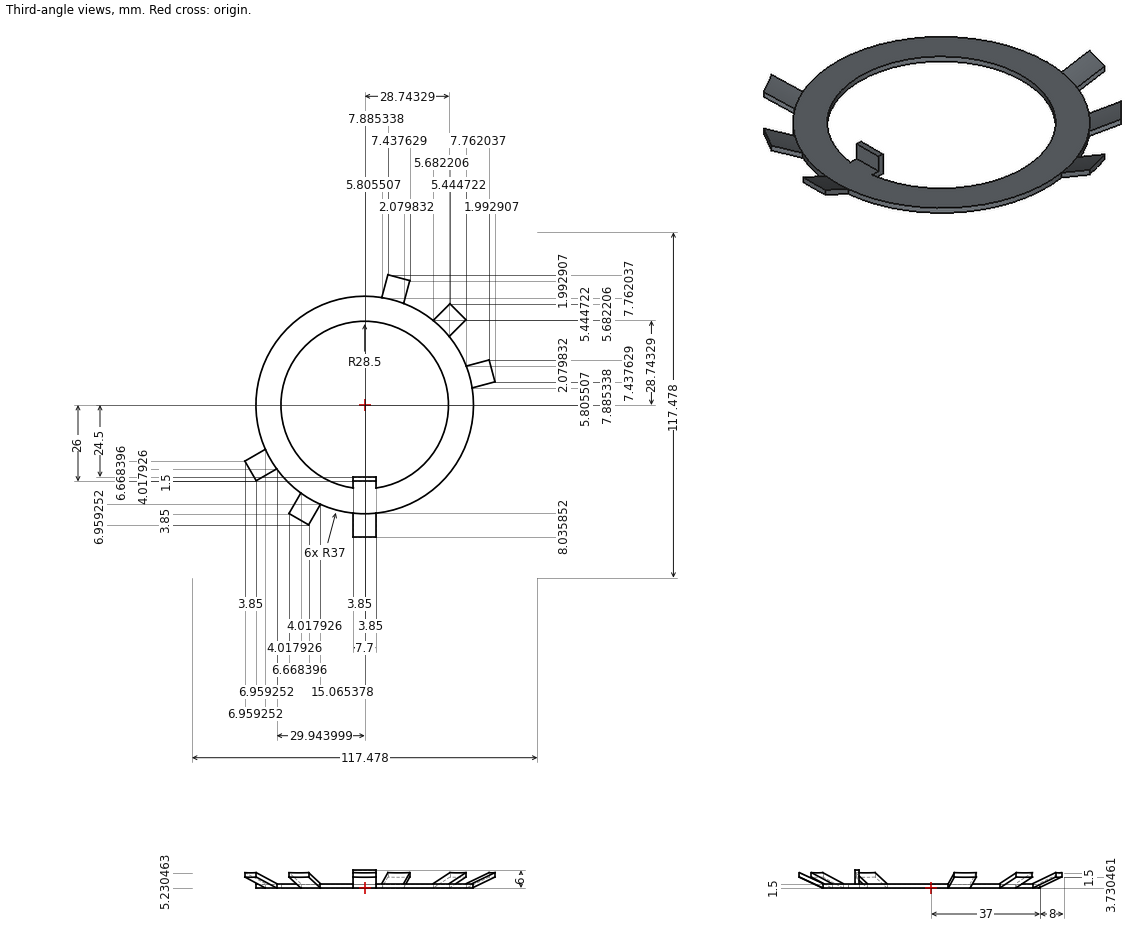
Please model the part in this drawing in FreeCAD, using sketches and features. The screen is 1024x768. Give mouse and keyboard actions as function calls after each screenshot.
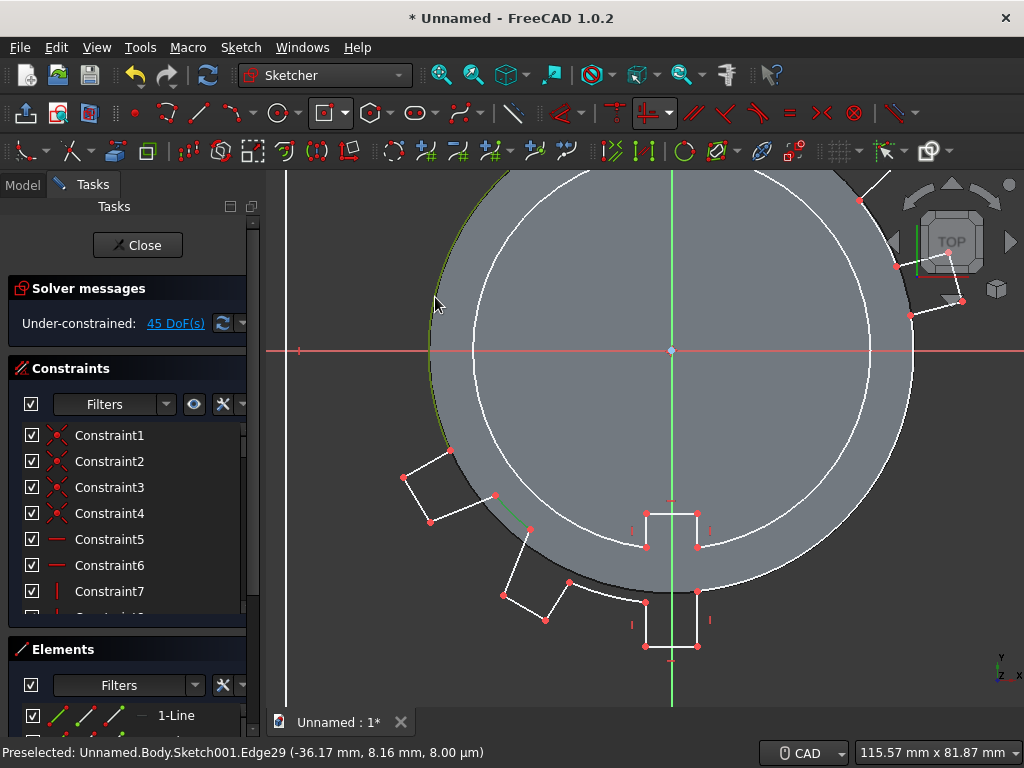
scroll(499, 510, down, 4)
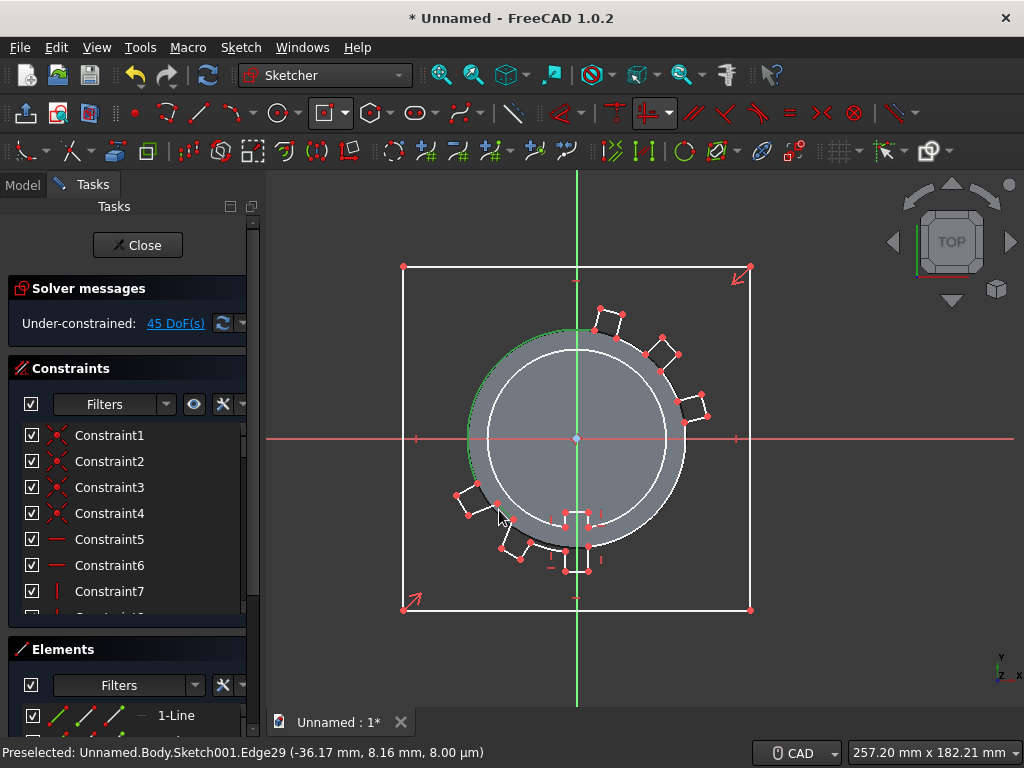
scroll(637, 349, up, 2)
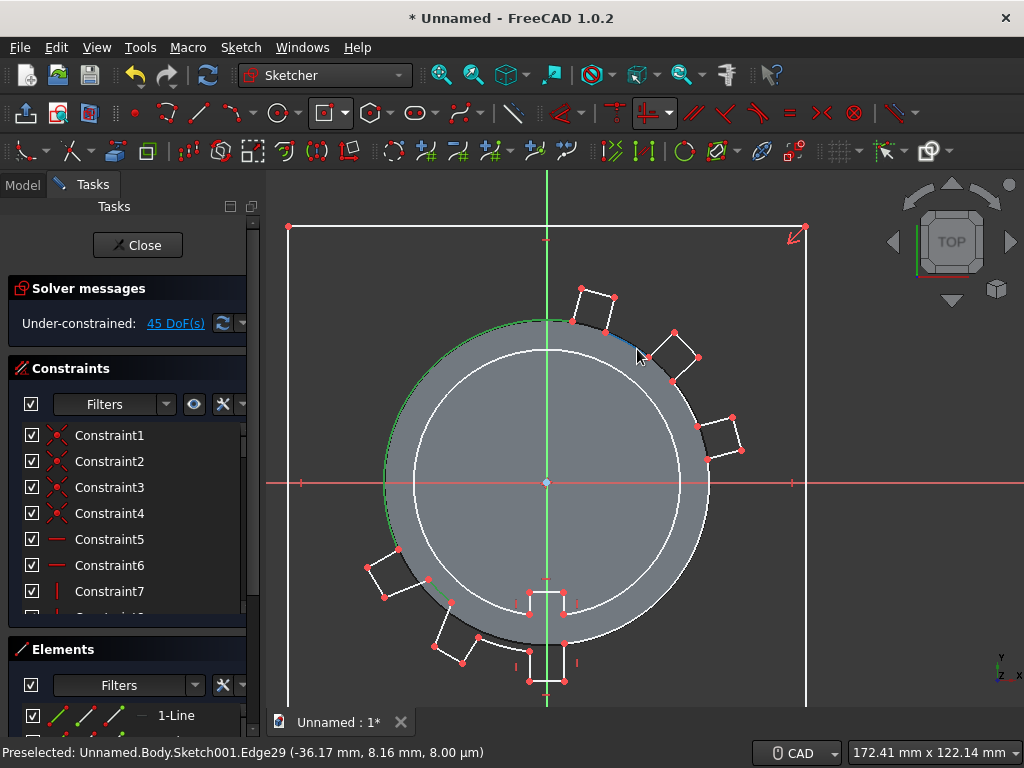
click(637, 349)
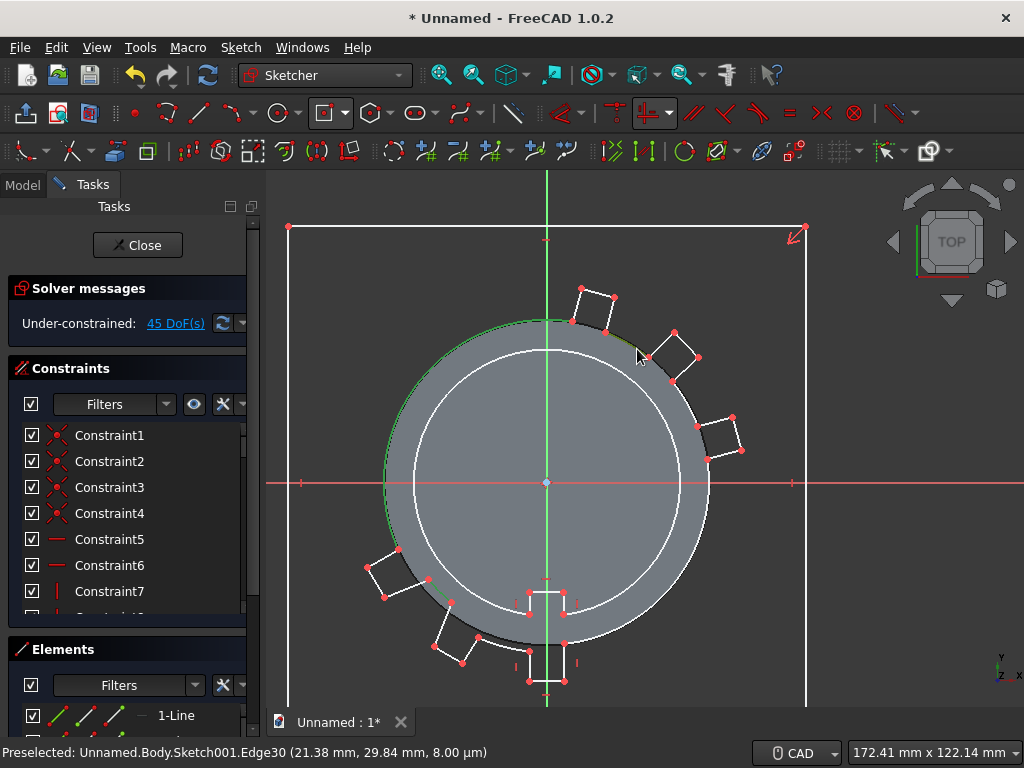
click(692, 412)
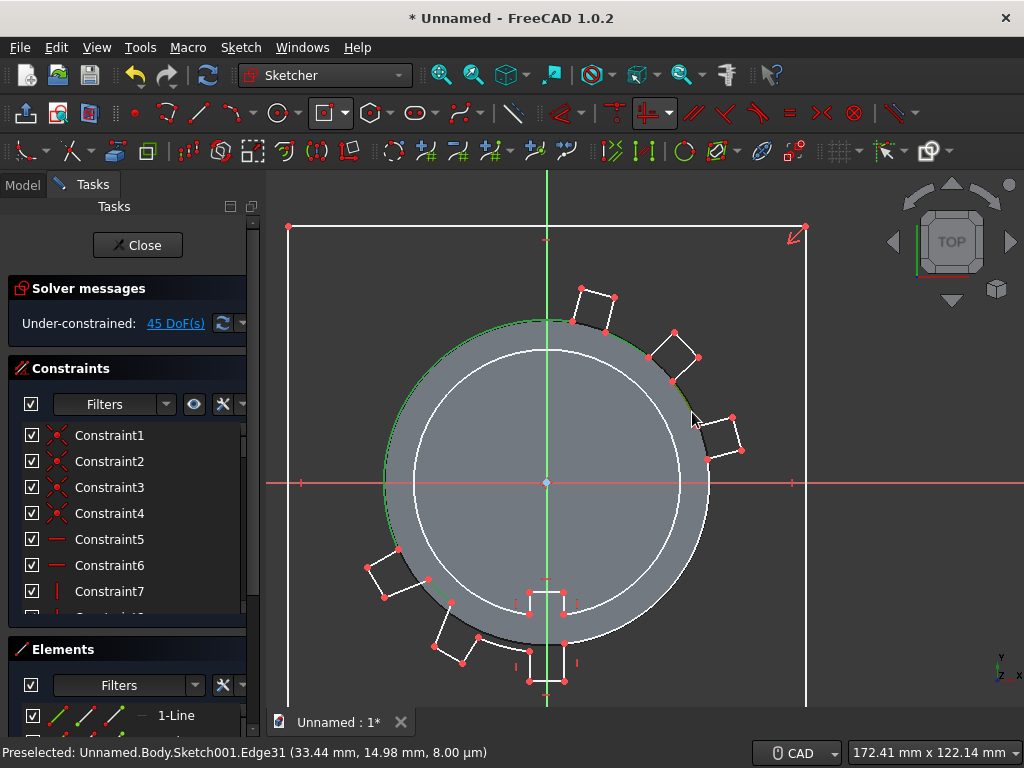
click(637, 617)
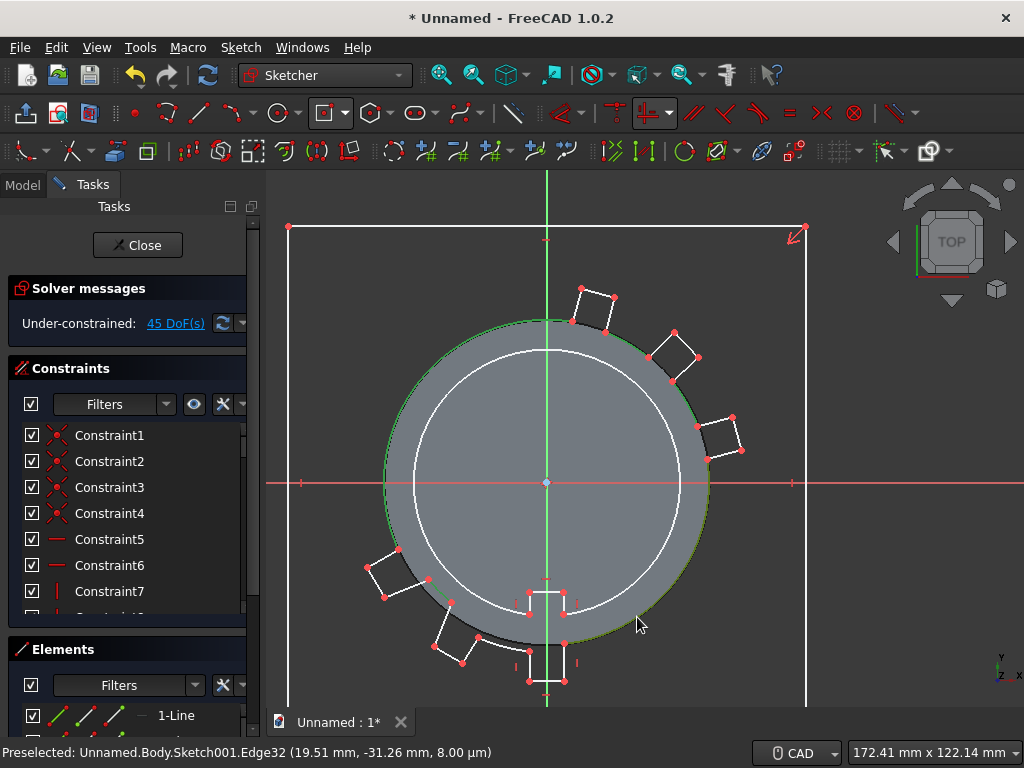
click(493, 644)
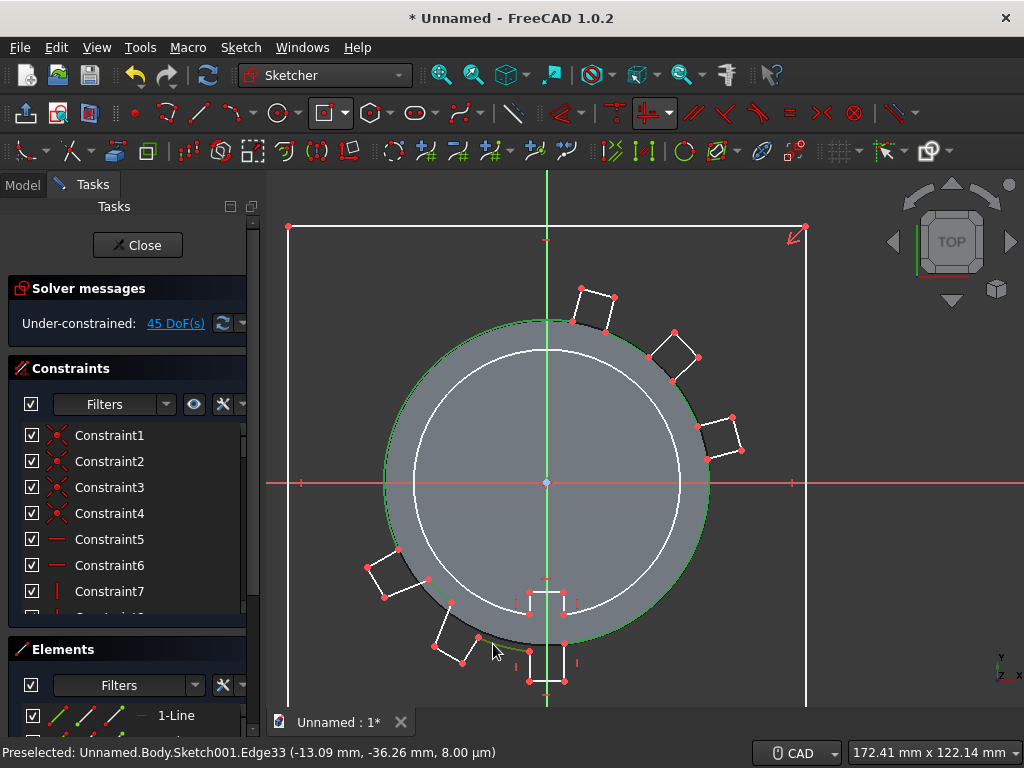
key(e)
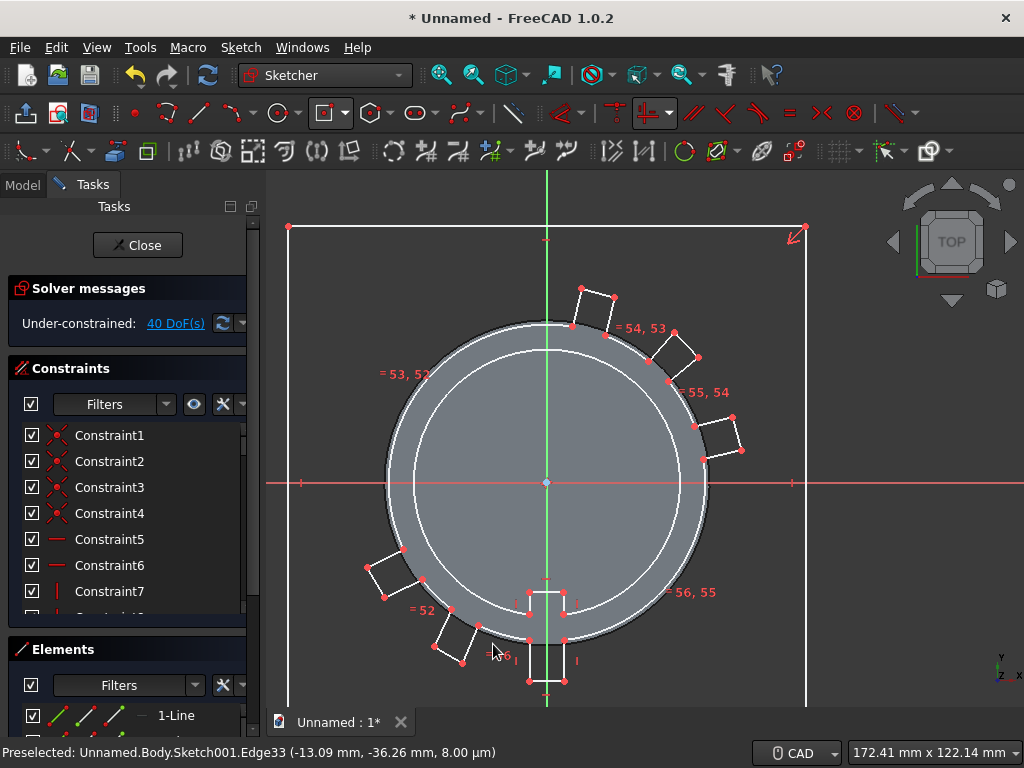
click(560, 114)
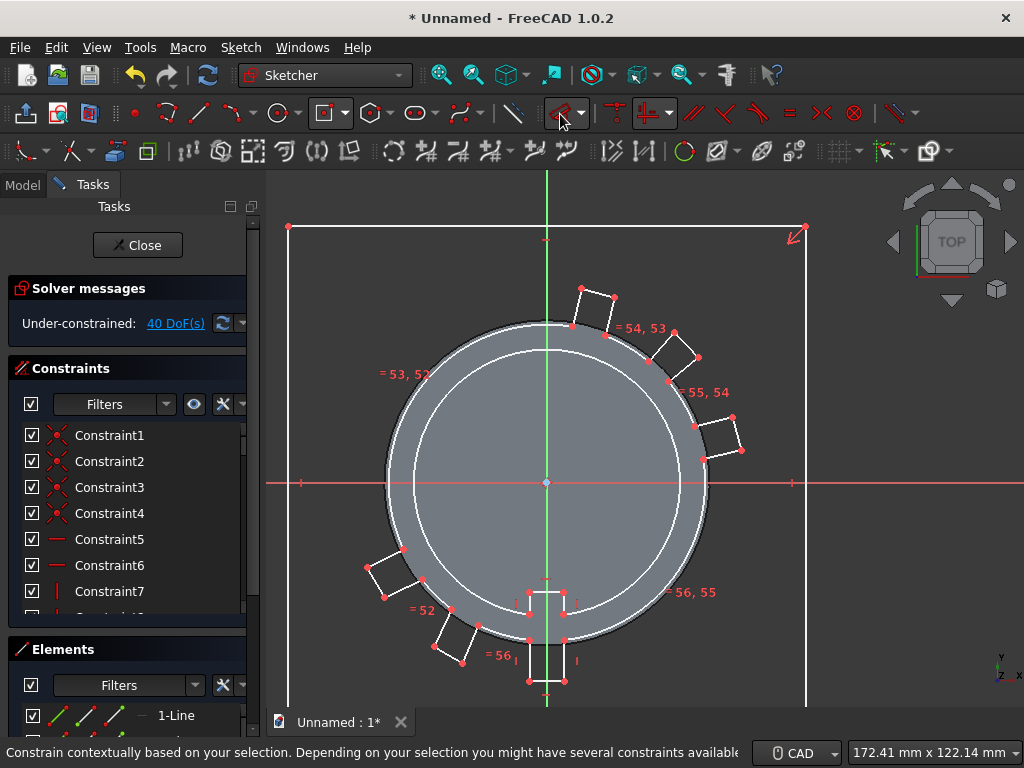
click(671, 435)
click(733, 508)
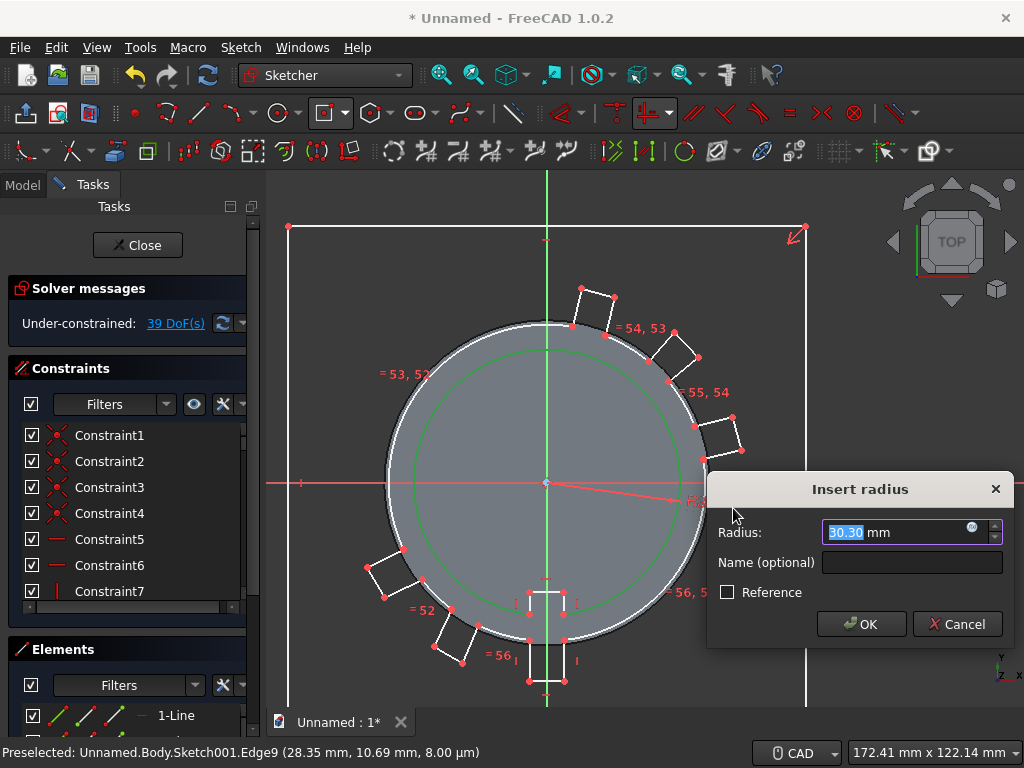
text(28.5)
key(Return)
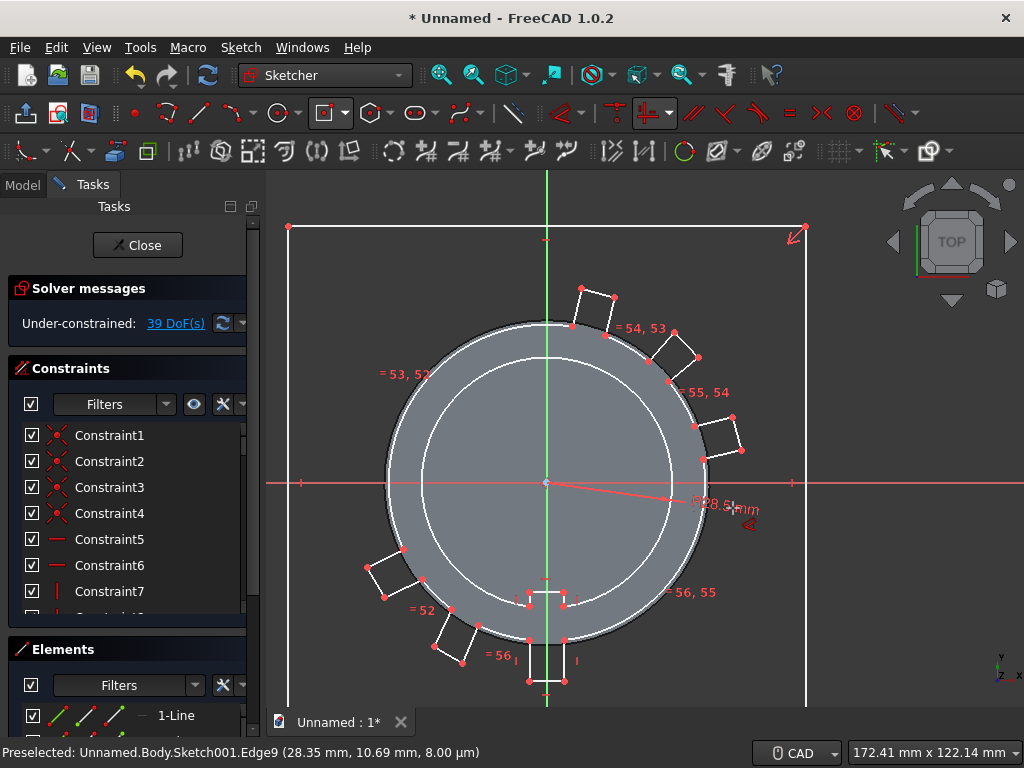
click(430, 590)
click(406, 612)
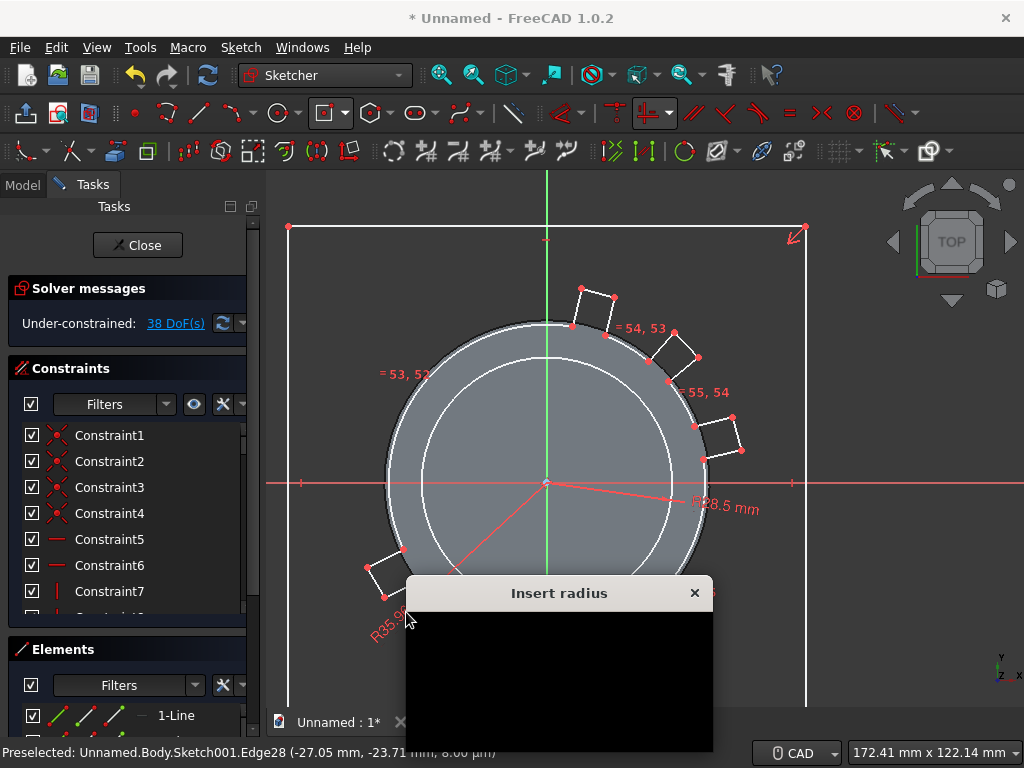
text(37)
key(Return)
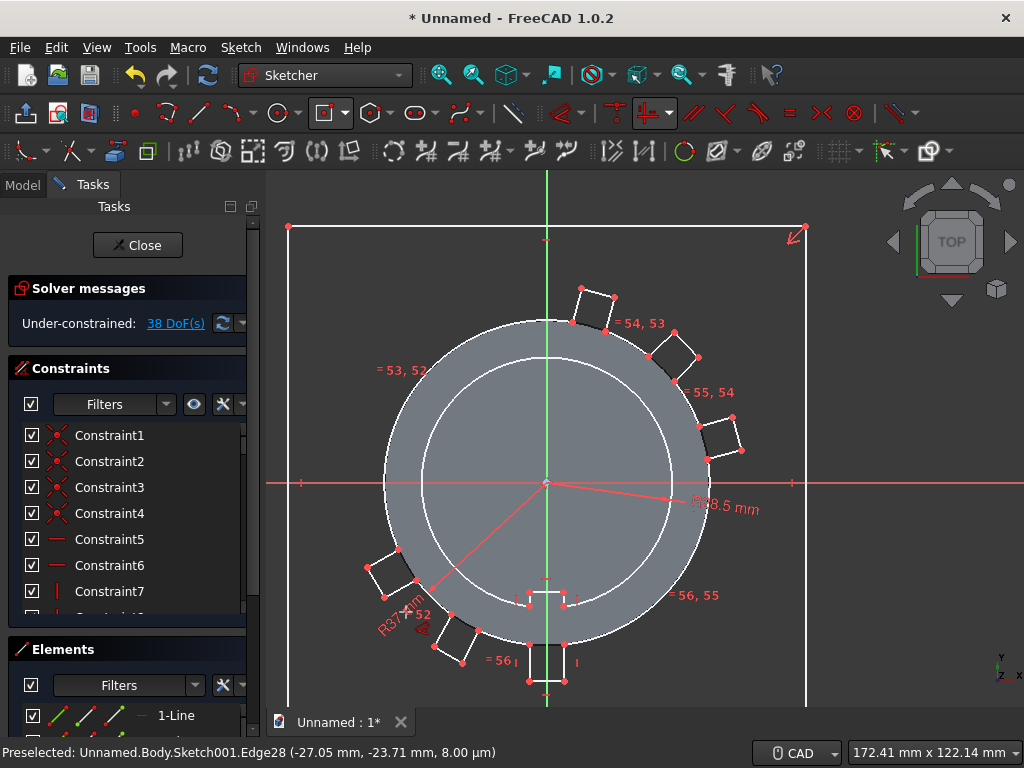
click(544, 592)
click(539, 626)